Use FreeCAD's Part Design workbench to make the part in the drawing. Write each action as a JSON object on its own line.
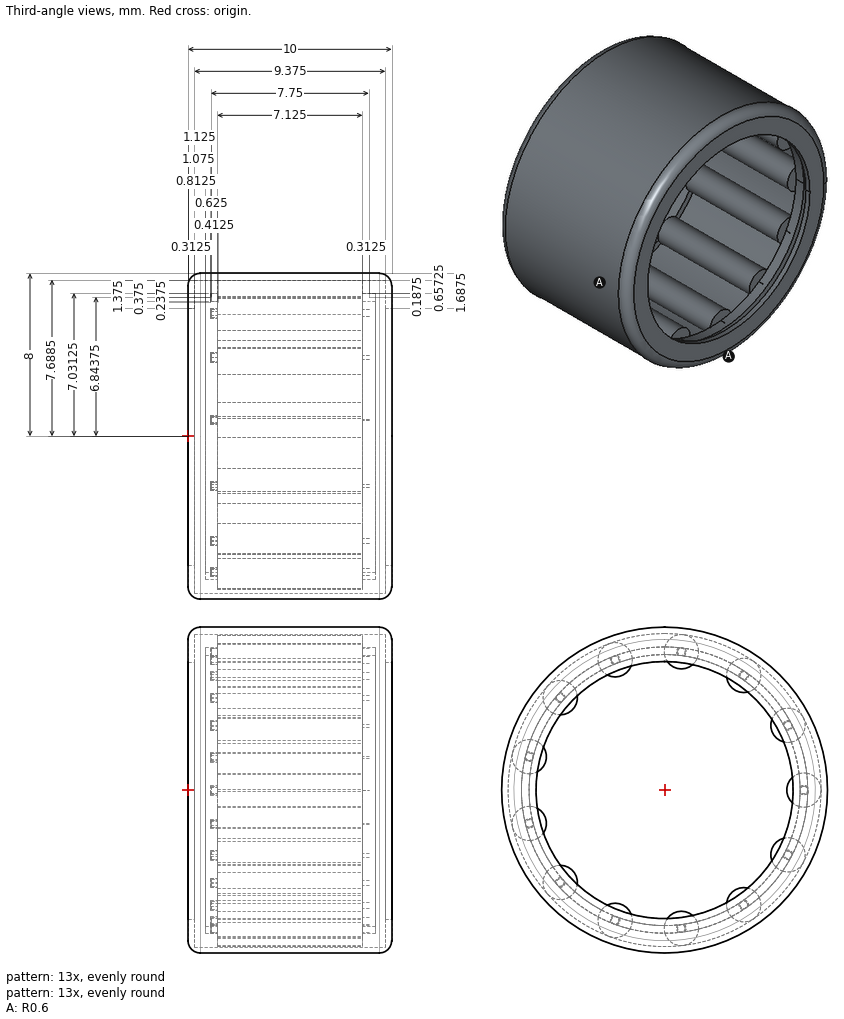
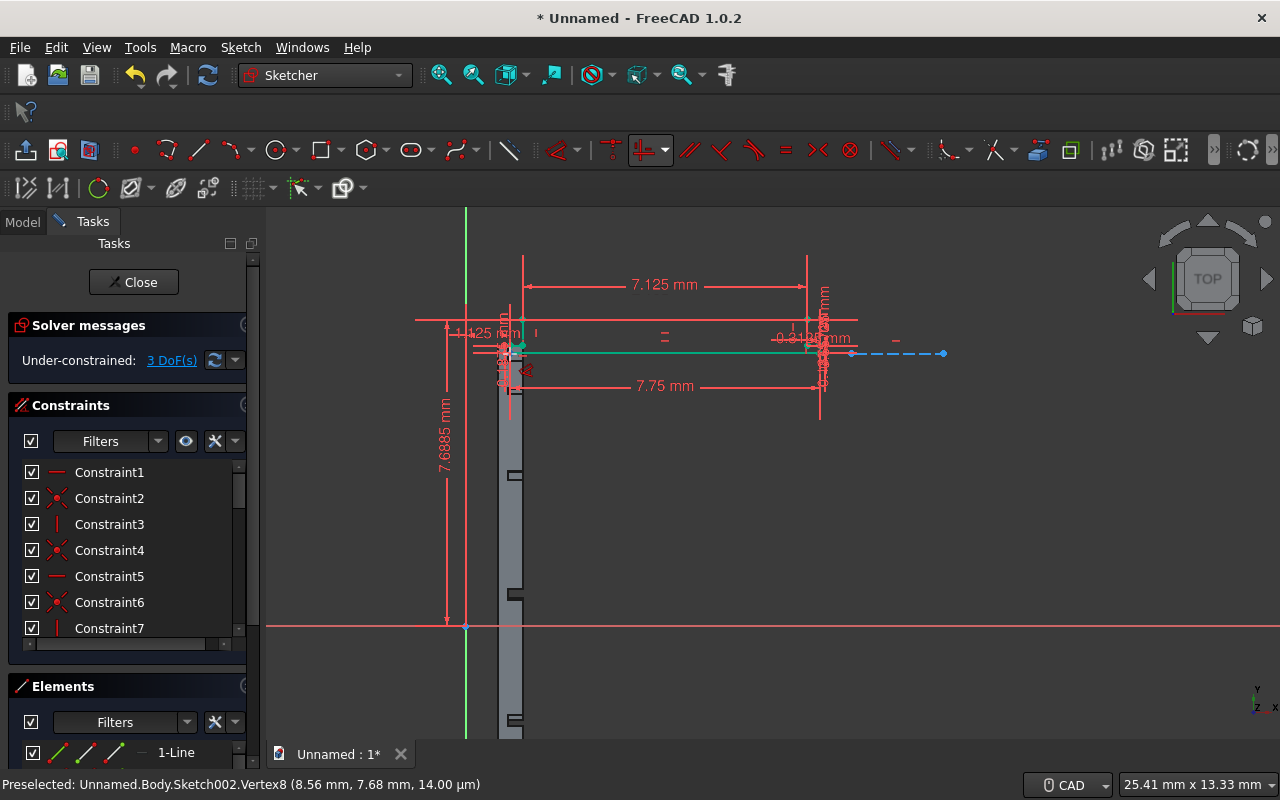
{"action": "left_click", "coordinate": [851, 354]}
{"action": "left_click", "coordinate": [432, 490]}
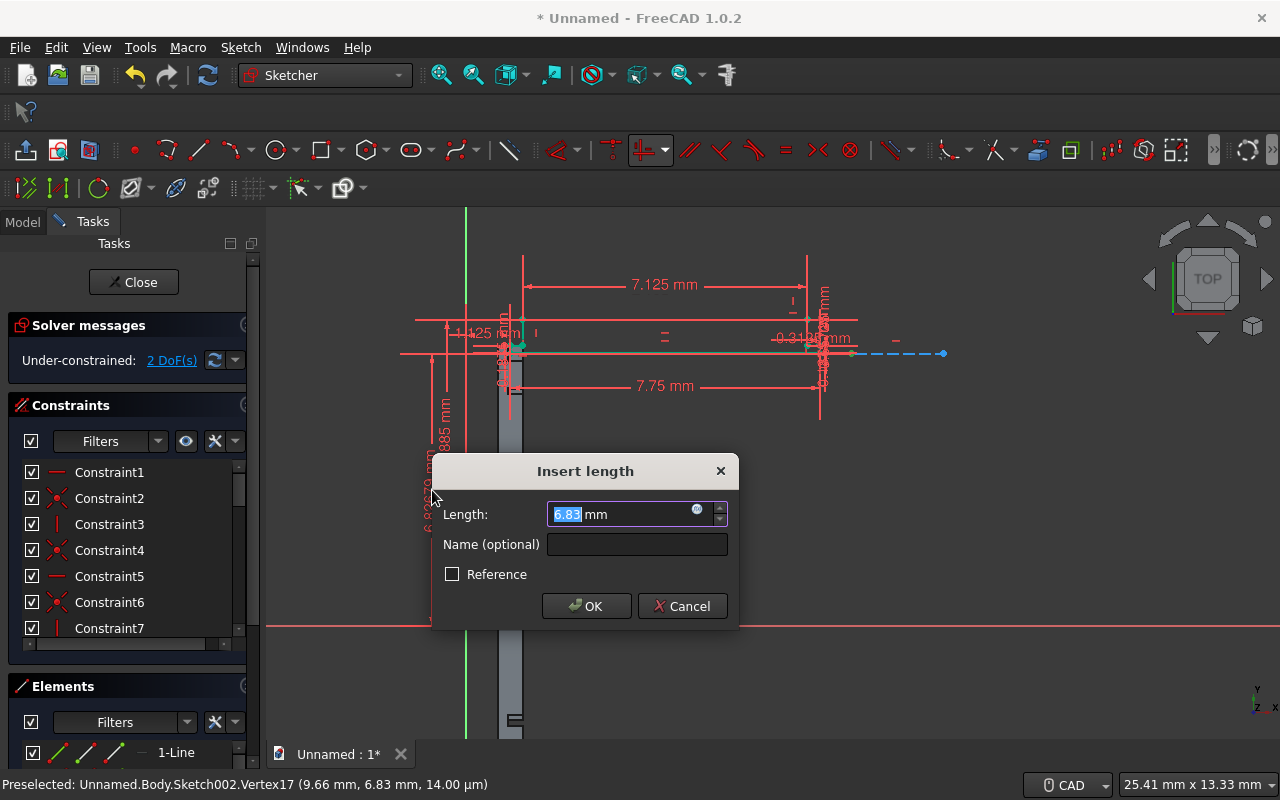
{"action": "type", "text": "6.84375"}
{"action": "key", "text": "Return"}
{"action": "key", "text": "Escape"}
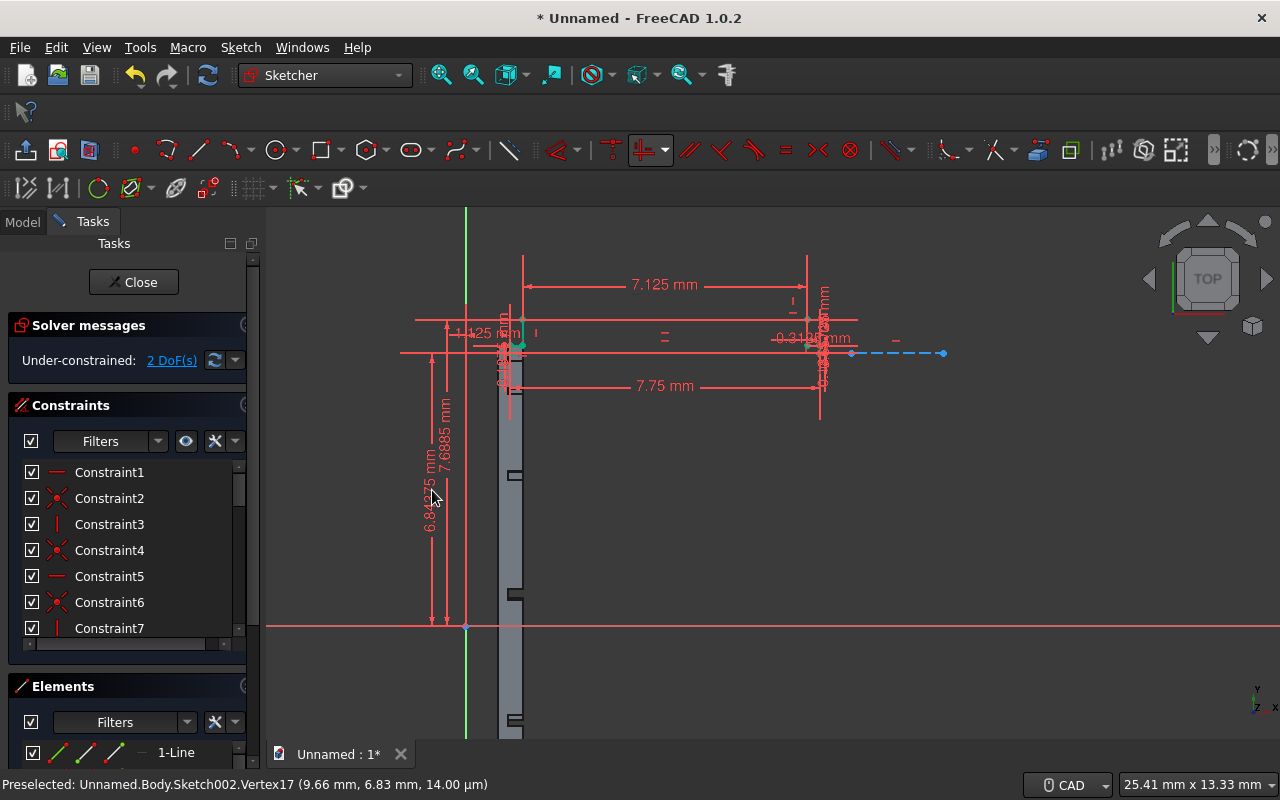
{"action": "left_click", "coordinate": [134, 282]}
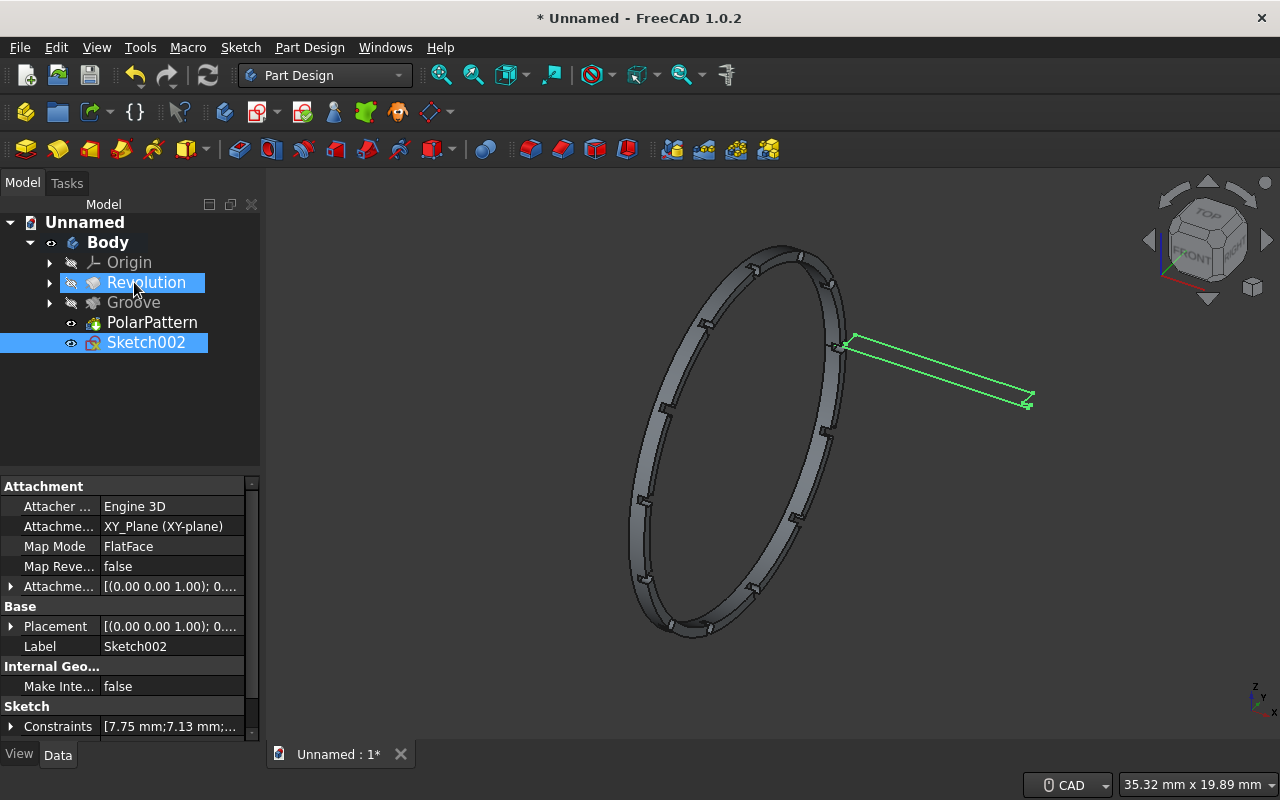
{"action": "left_click", "coordinate": [58, 150]}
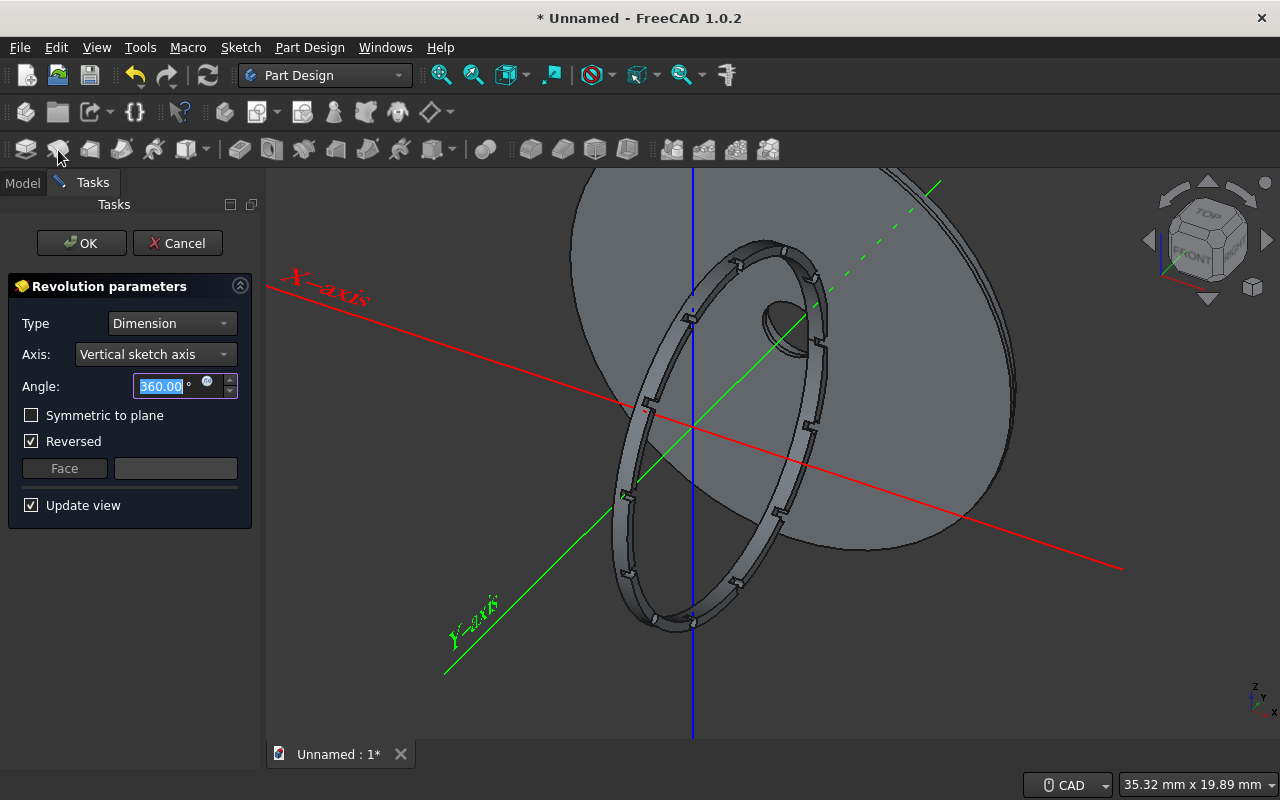
{"action": "left_click", "coordinate": [156, 354]}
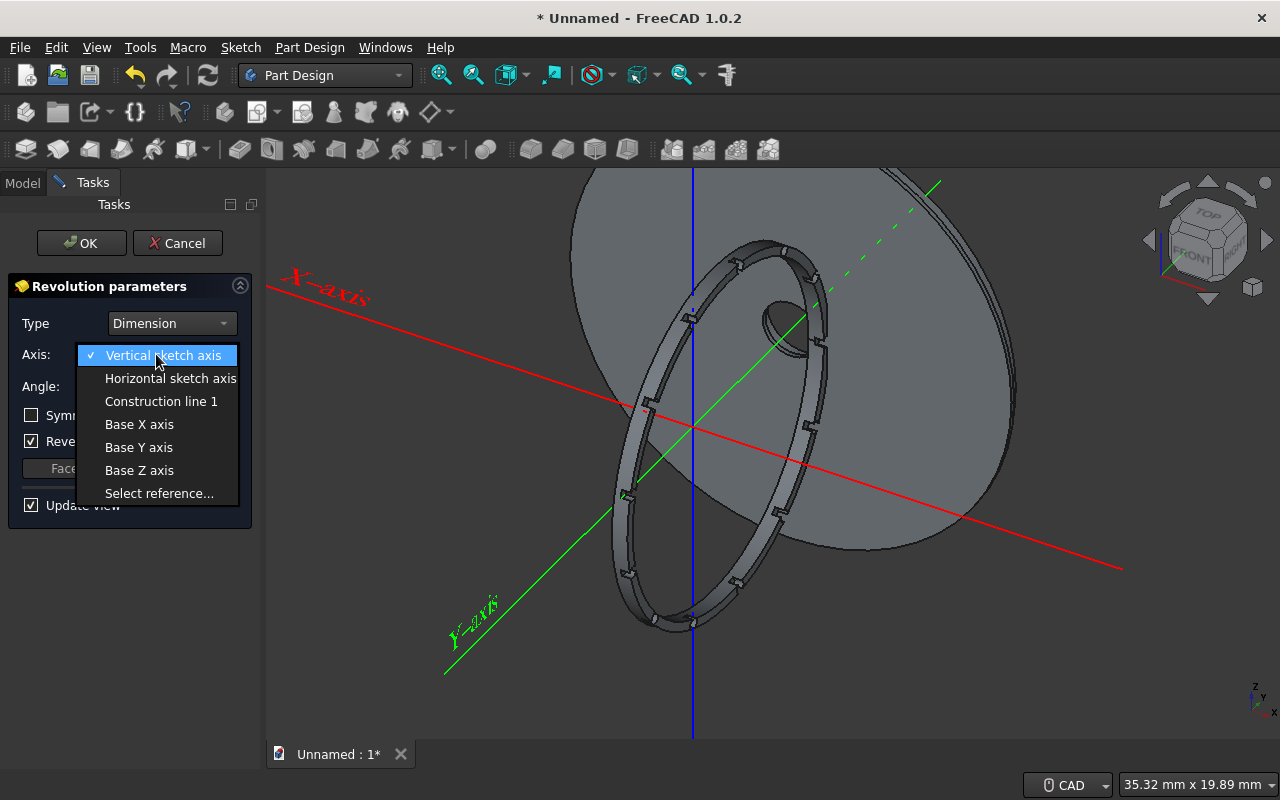
{"action": "left_click", "coordinate": [156, 402]}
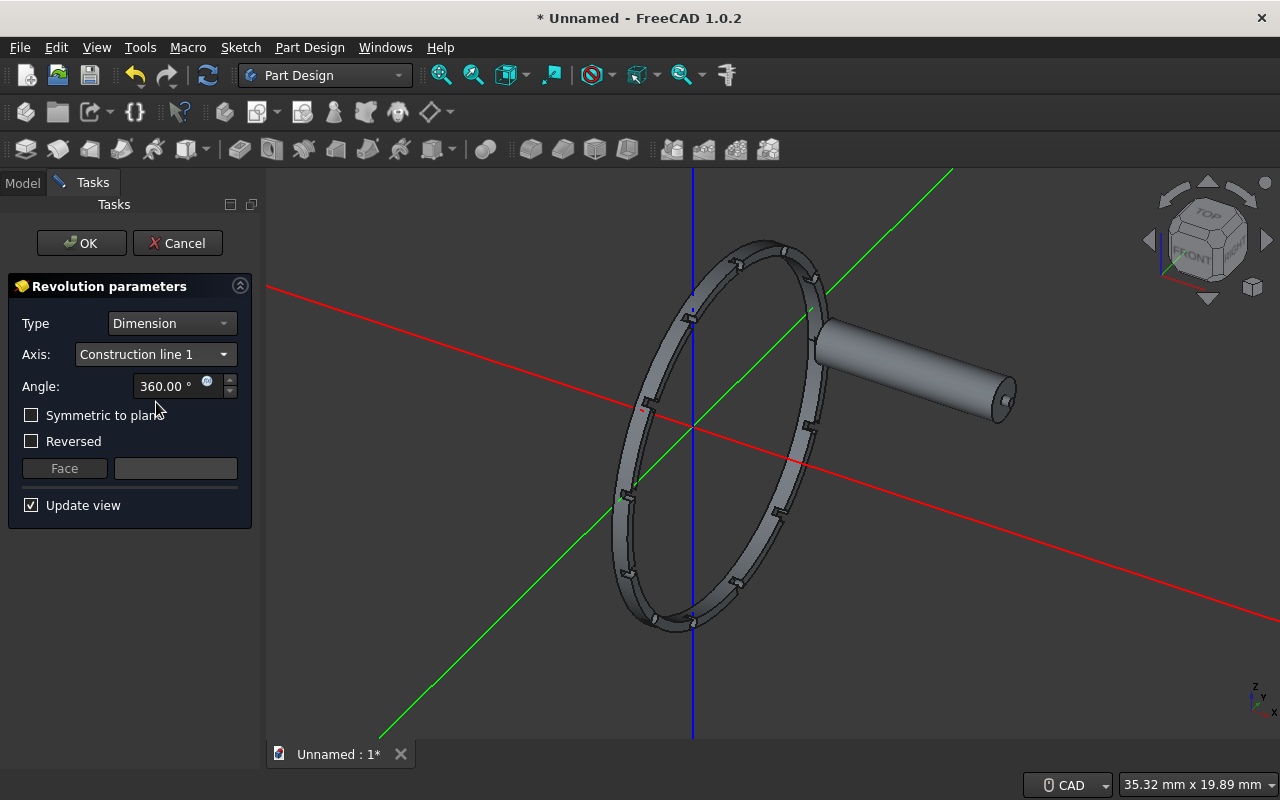
{"action": "left_click", "coordinate": [82, 243]}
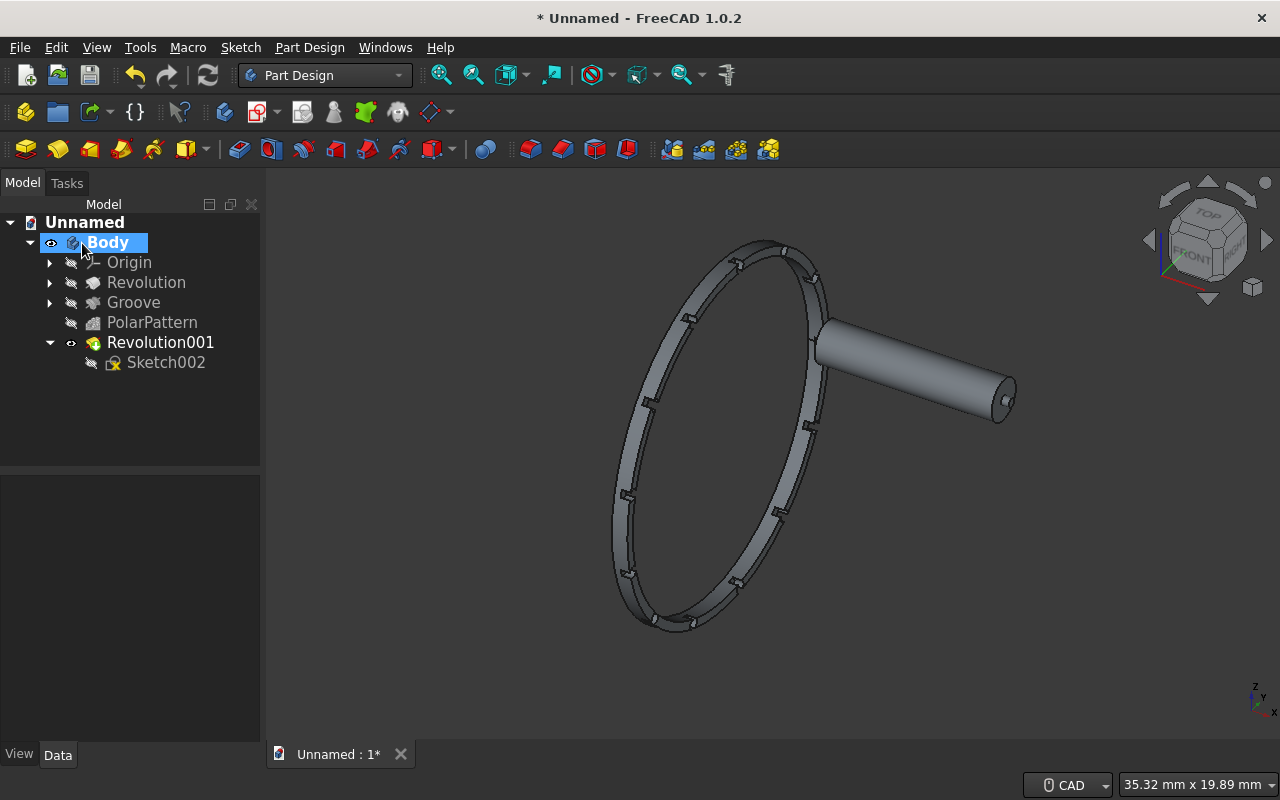
{"action": "left_click", "coordinate": [442, 76]}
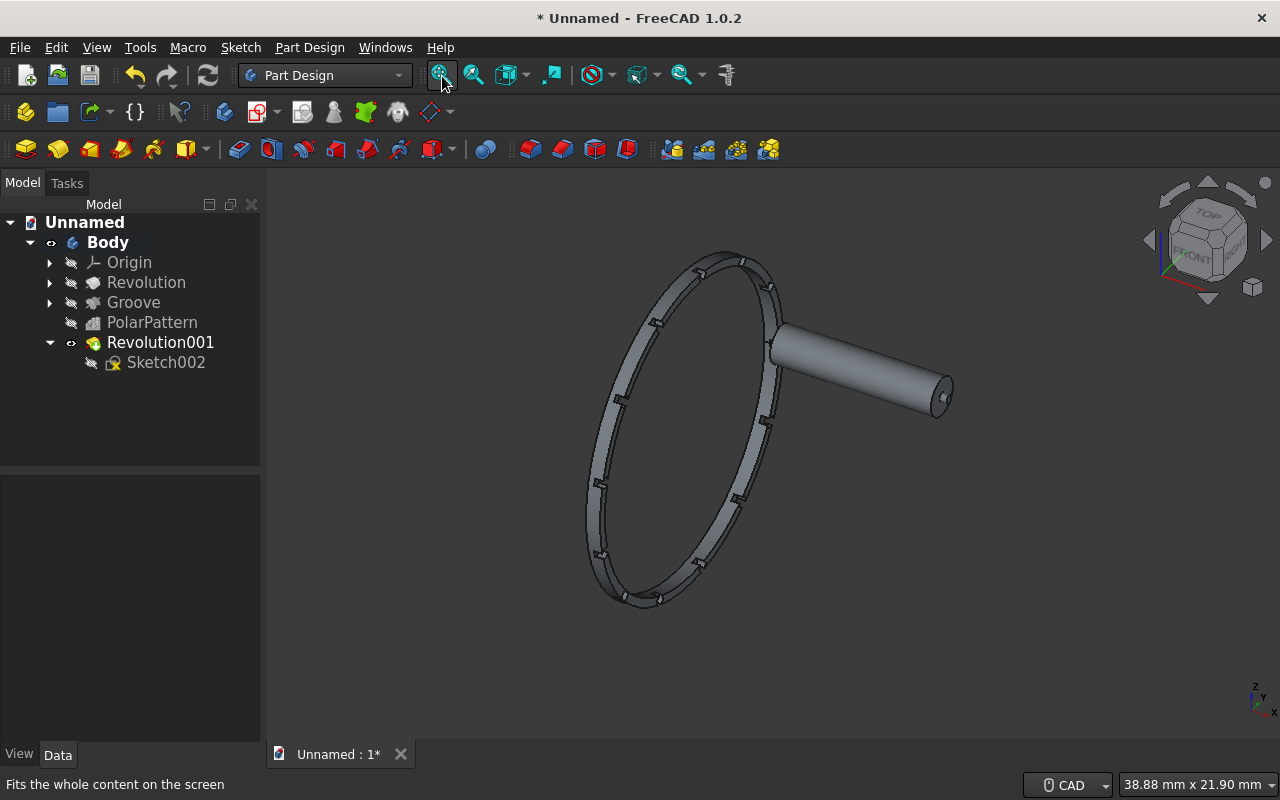
{"action": "left_click", "coordinate": [258, 112]}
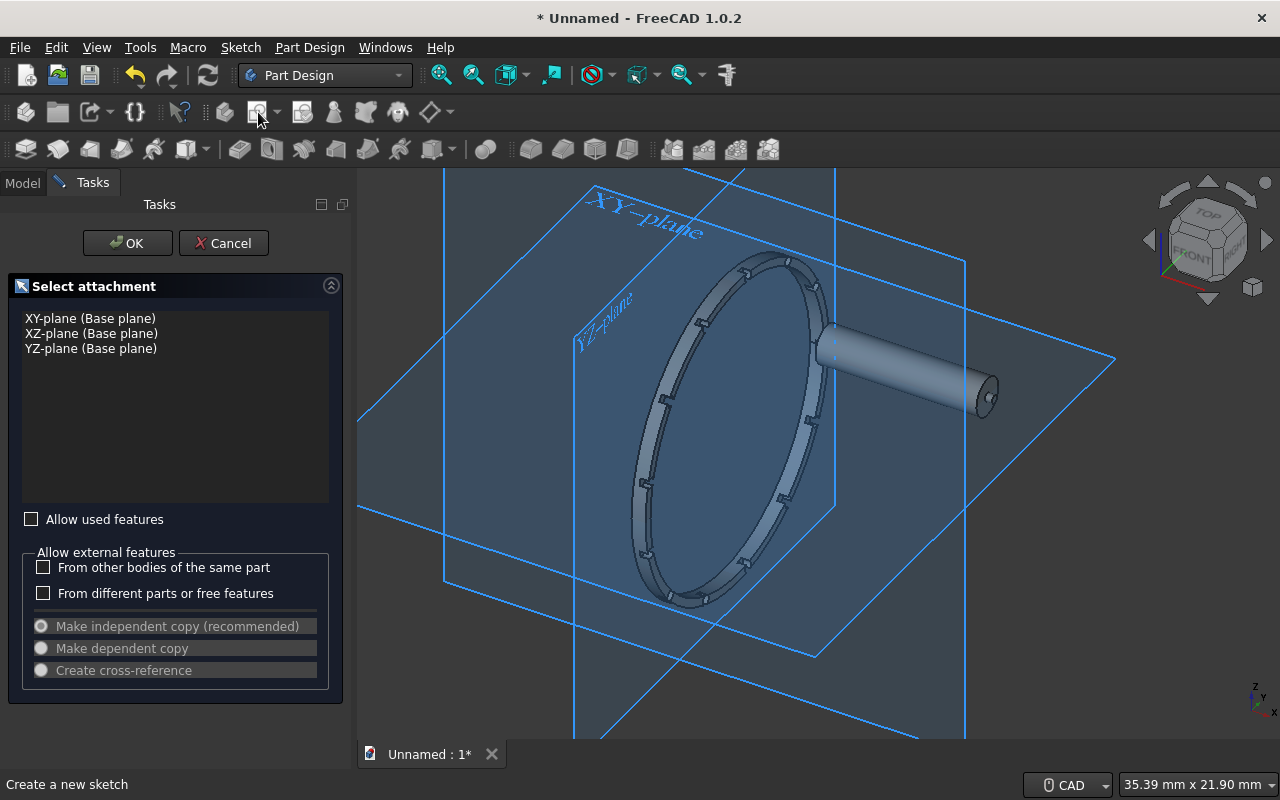
{"action": "left_click", "coordinate": [82, 318]}